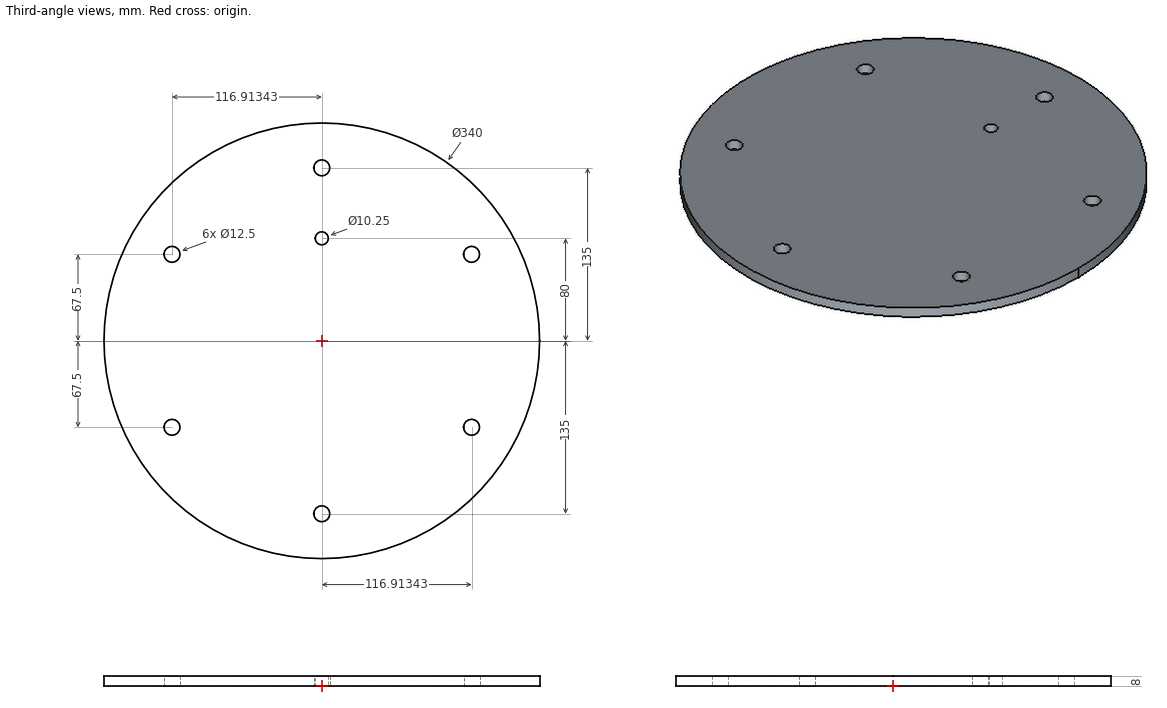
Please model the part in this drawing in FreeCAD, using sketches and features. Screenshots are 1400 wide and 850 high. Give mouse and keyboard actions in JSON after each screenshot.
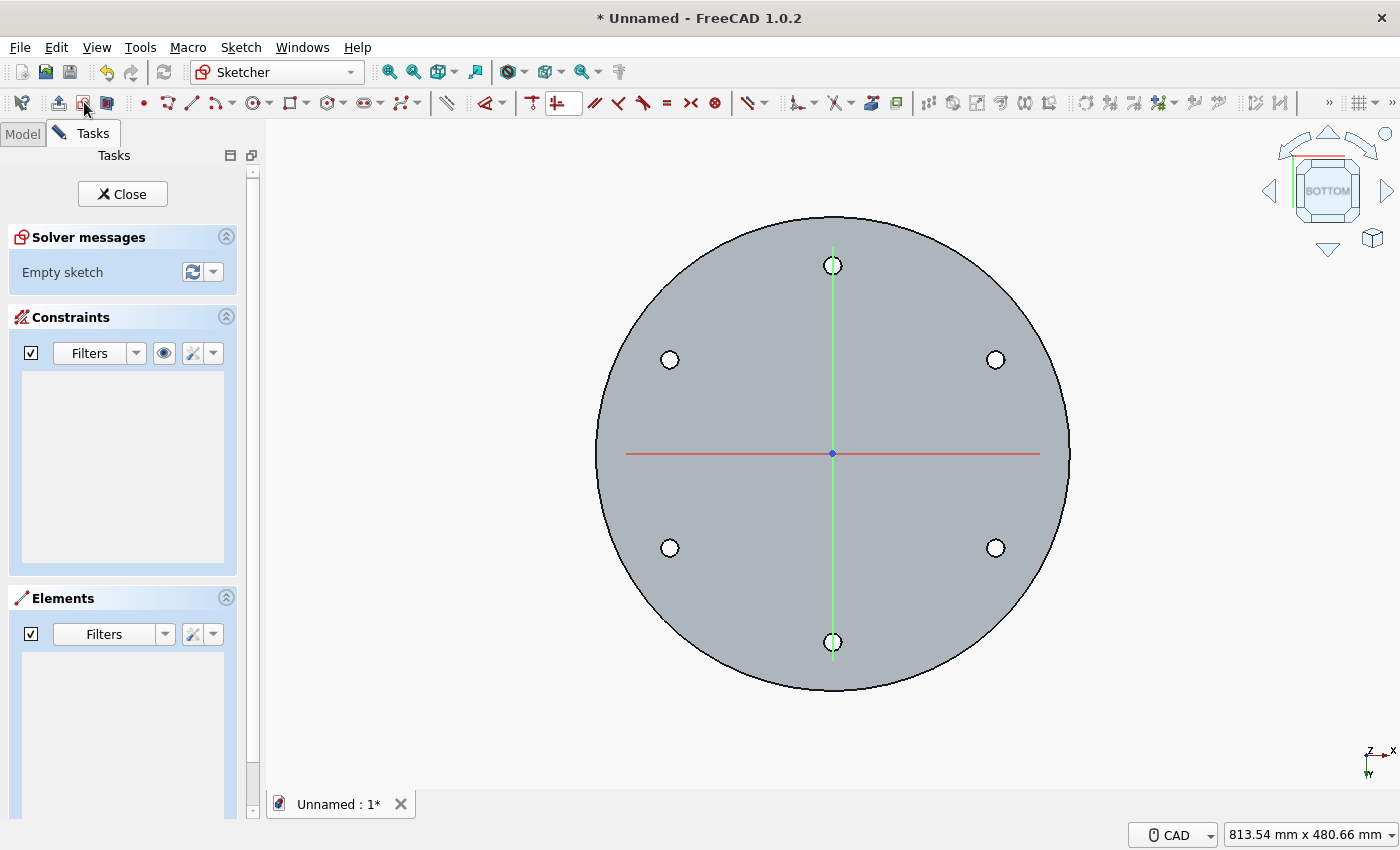
{"action": "scroll", "coordinate": [836, 571], "scroll_direction": "up", "scroll_amount": 15}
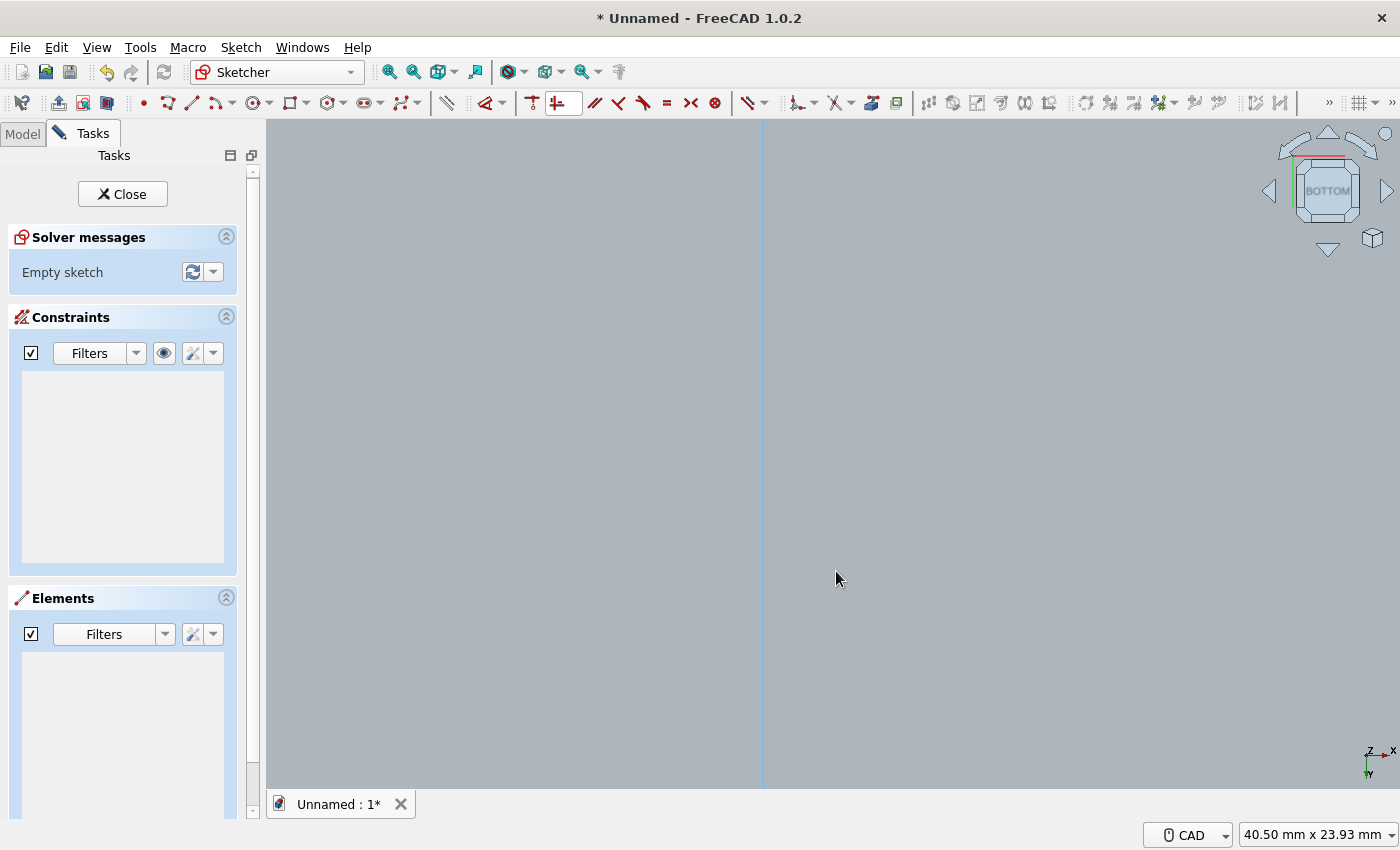
{"action": "scroll", "coordinate": [760, 436], "scroll_direction": "up", "scroll_amount": 2}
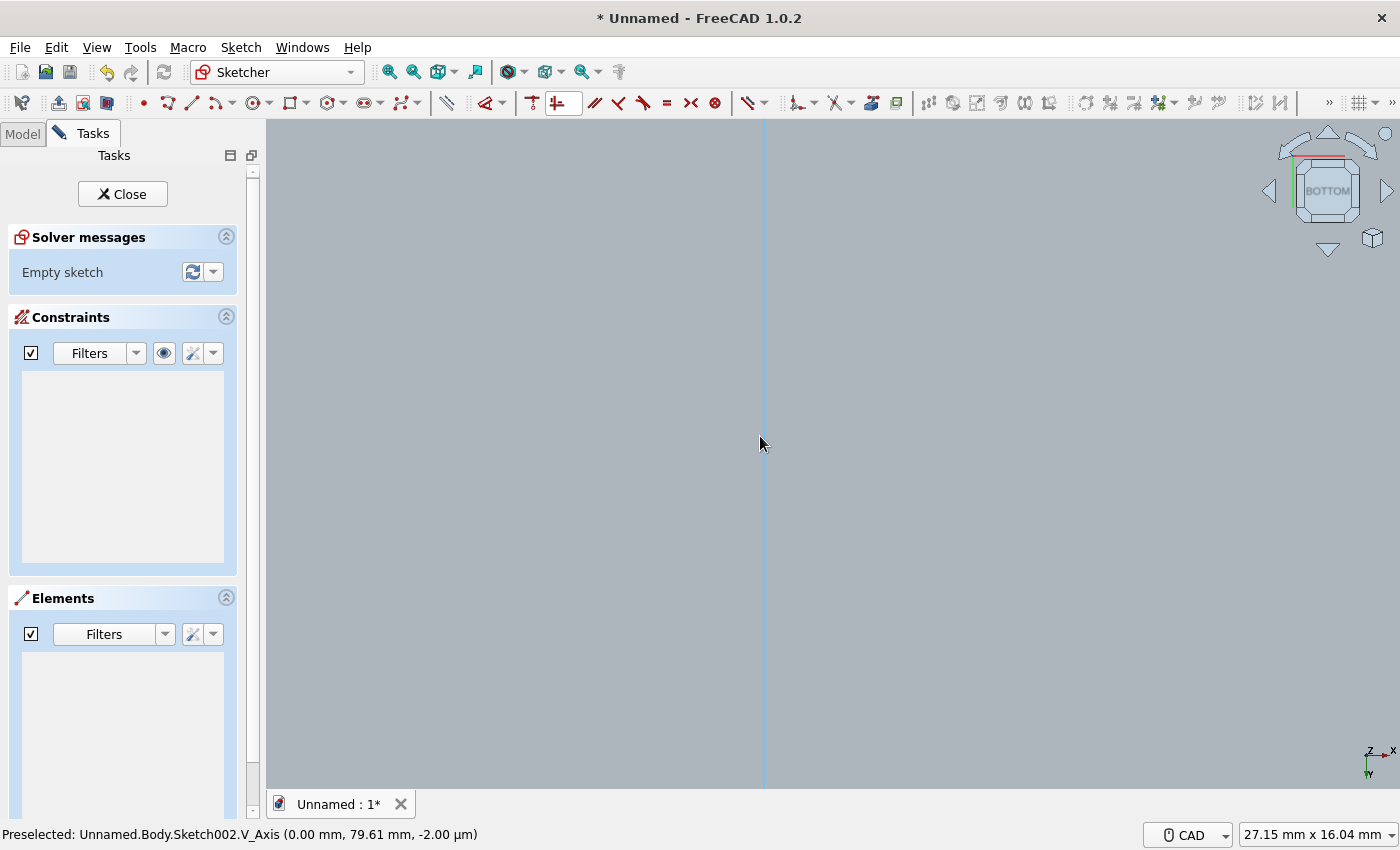
{"action": "left_click", "coordinate": [254, 104]}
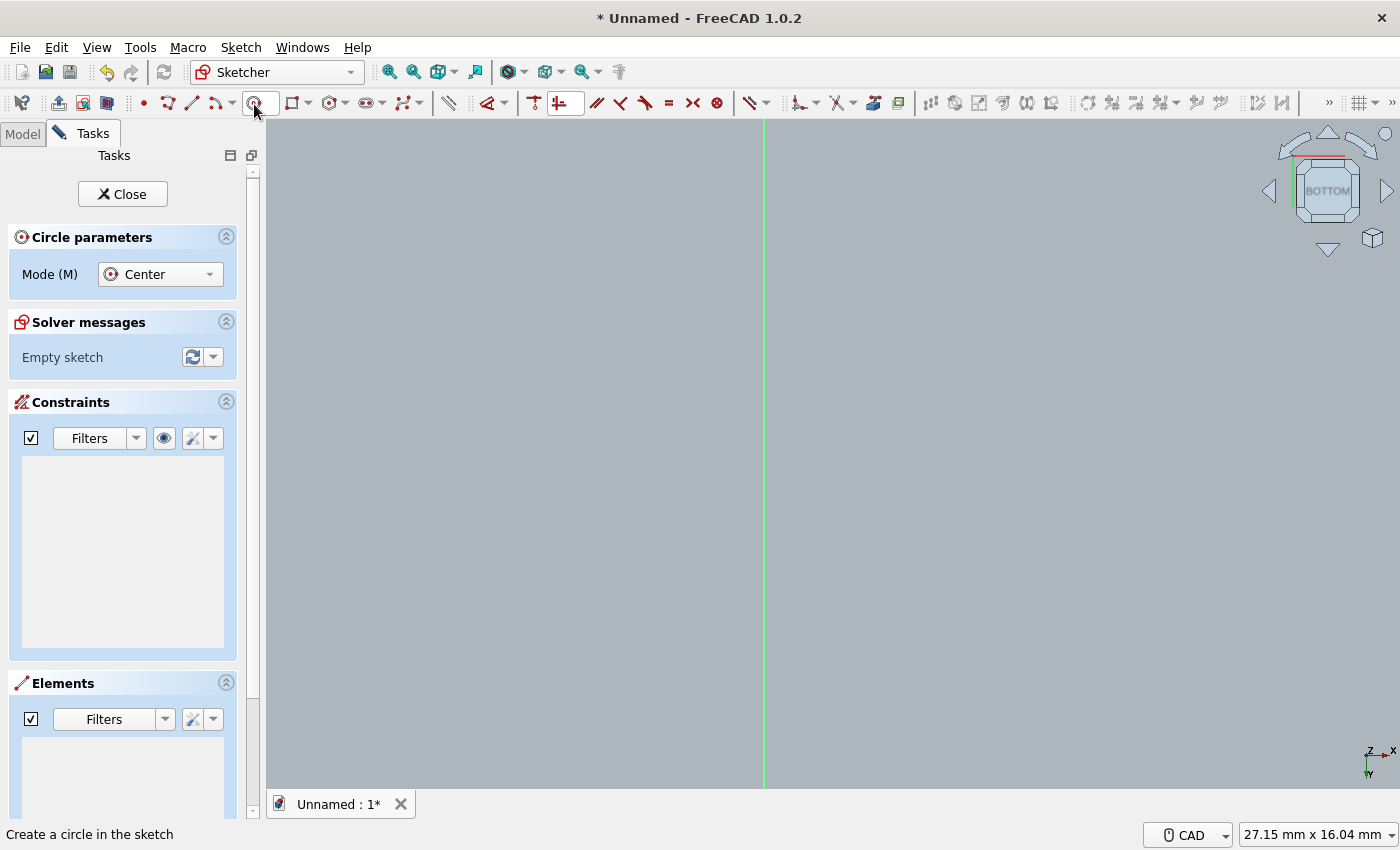
{"action": "left_click", "coordinate": [764, 454]}
{"action": "mouse_move", "coordinate": [916, 302]}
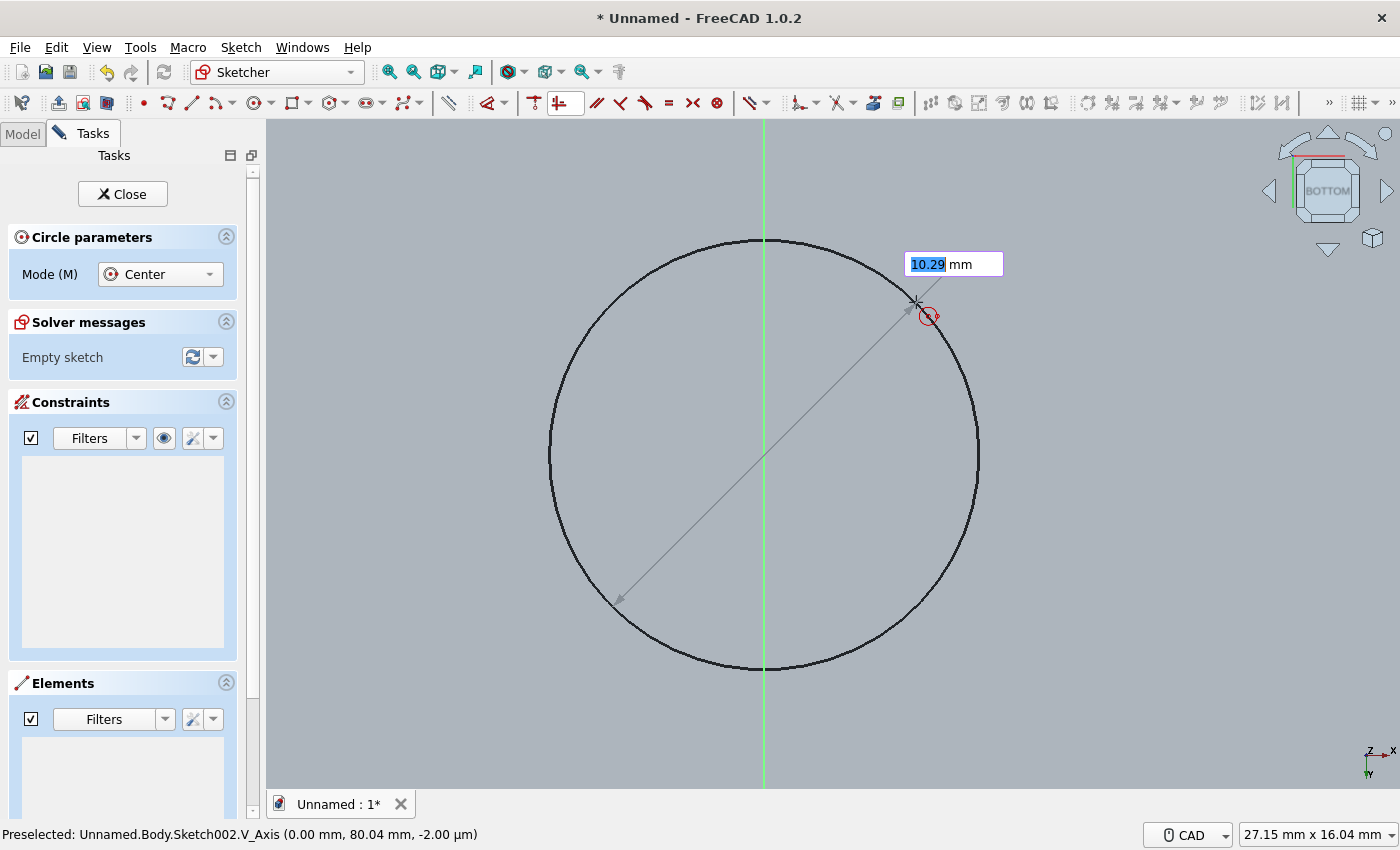
{"action": "type", "text": "10.25"}
{"action": "key", "text": "Return"}
{"action": "key", "text": "Escape"}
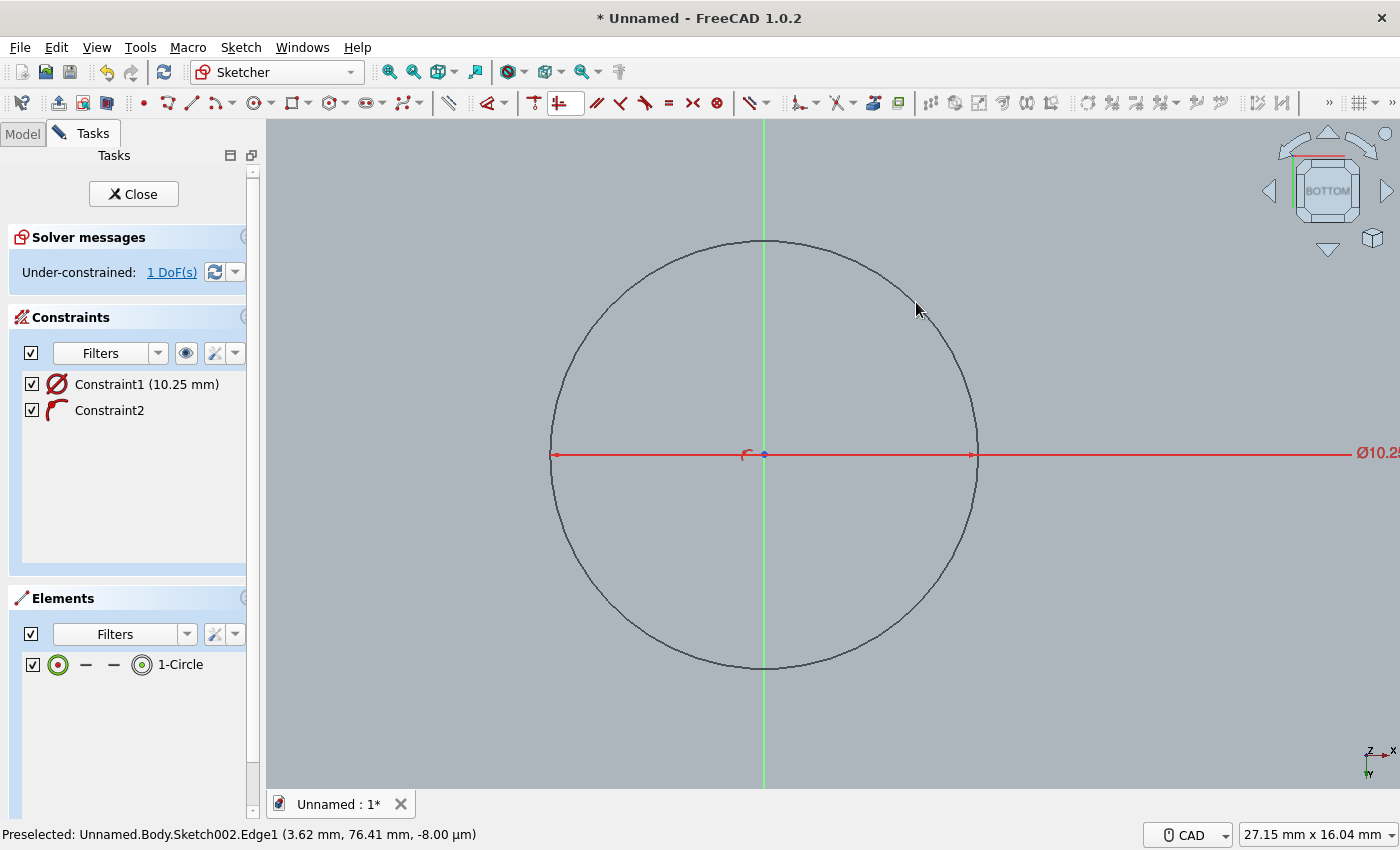
{"action": "left_click", "coordinate": [488, 104]}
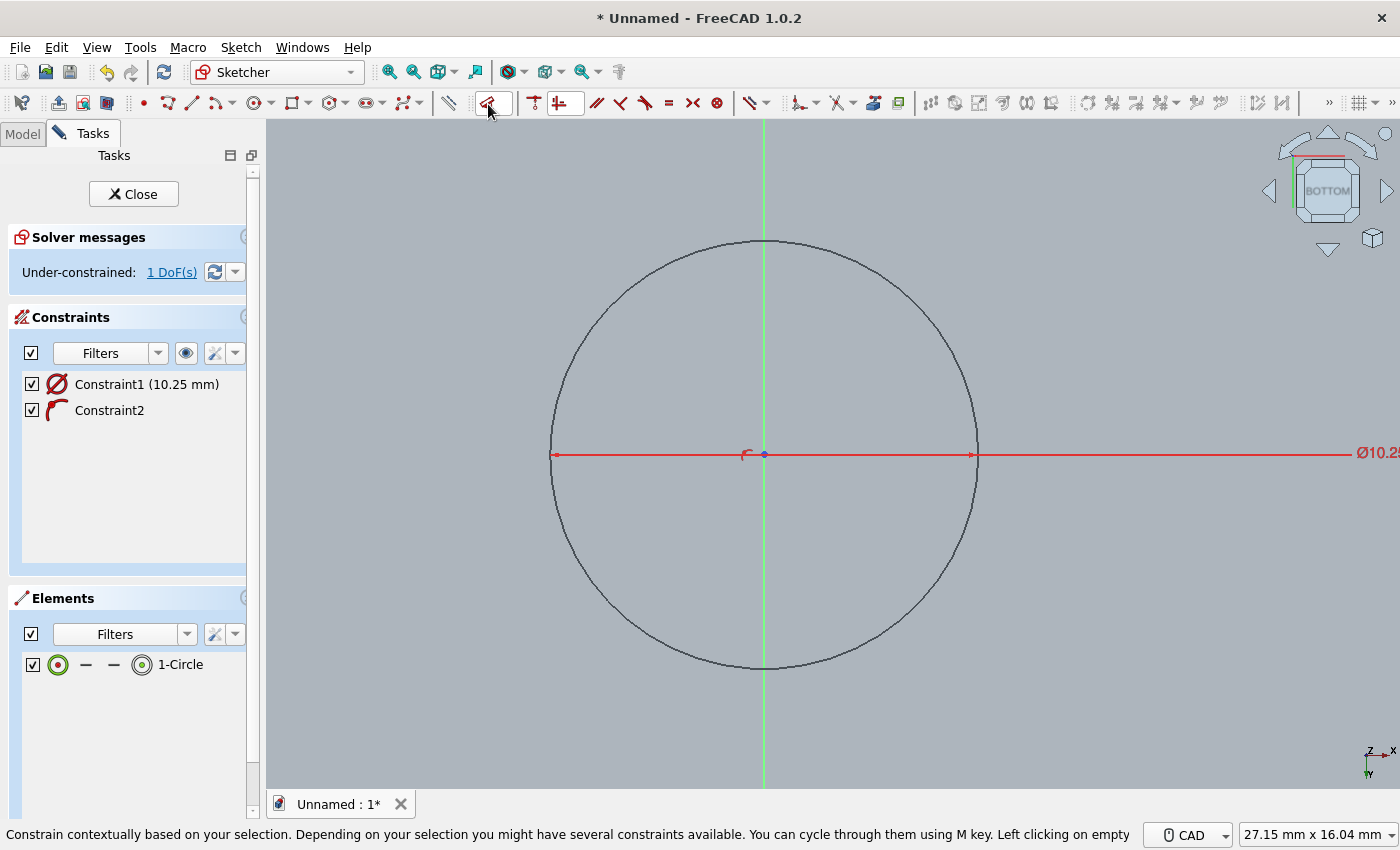
{"action": "left_click", "coordinate": [764, 455]}
{"action": "left_click", "coordinate": [798, 301]}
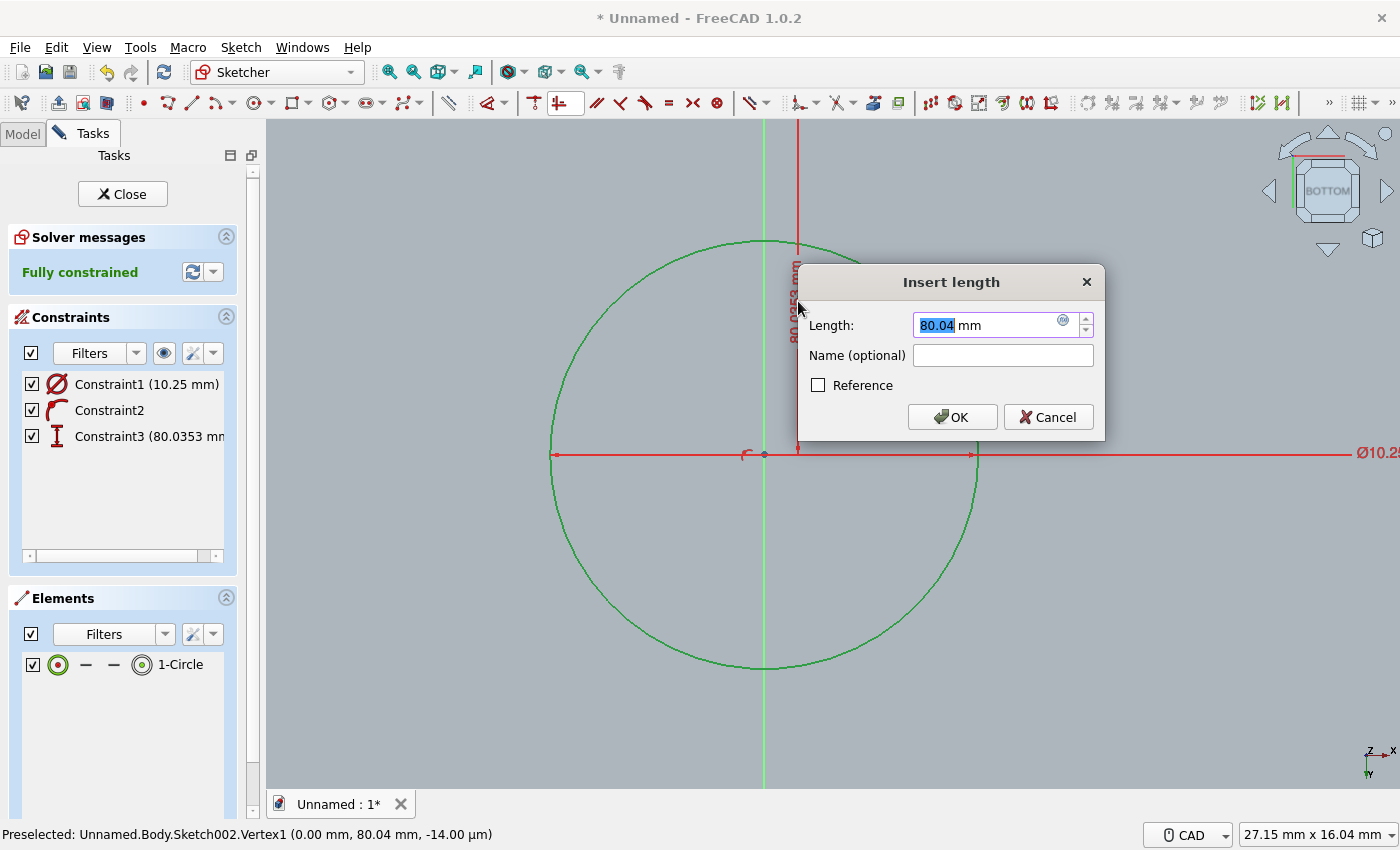
{"action": "type", "text": "80"}
{"action": "key", "text": "Return"}
{"action": "key", "text": "Escape"}